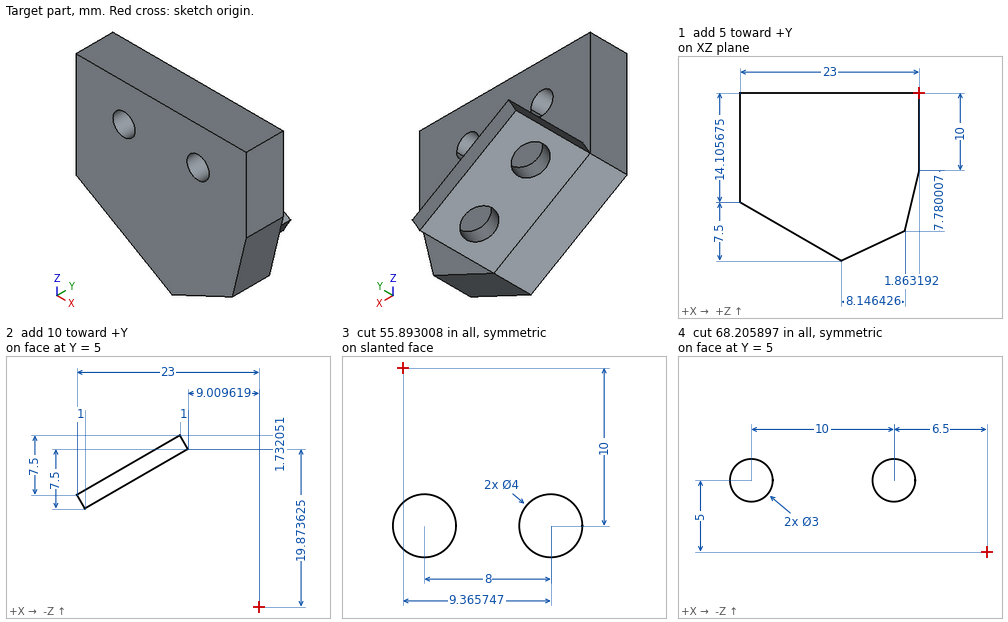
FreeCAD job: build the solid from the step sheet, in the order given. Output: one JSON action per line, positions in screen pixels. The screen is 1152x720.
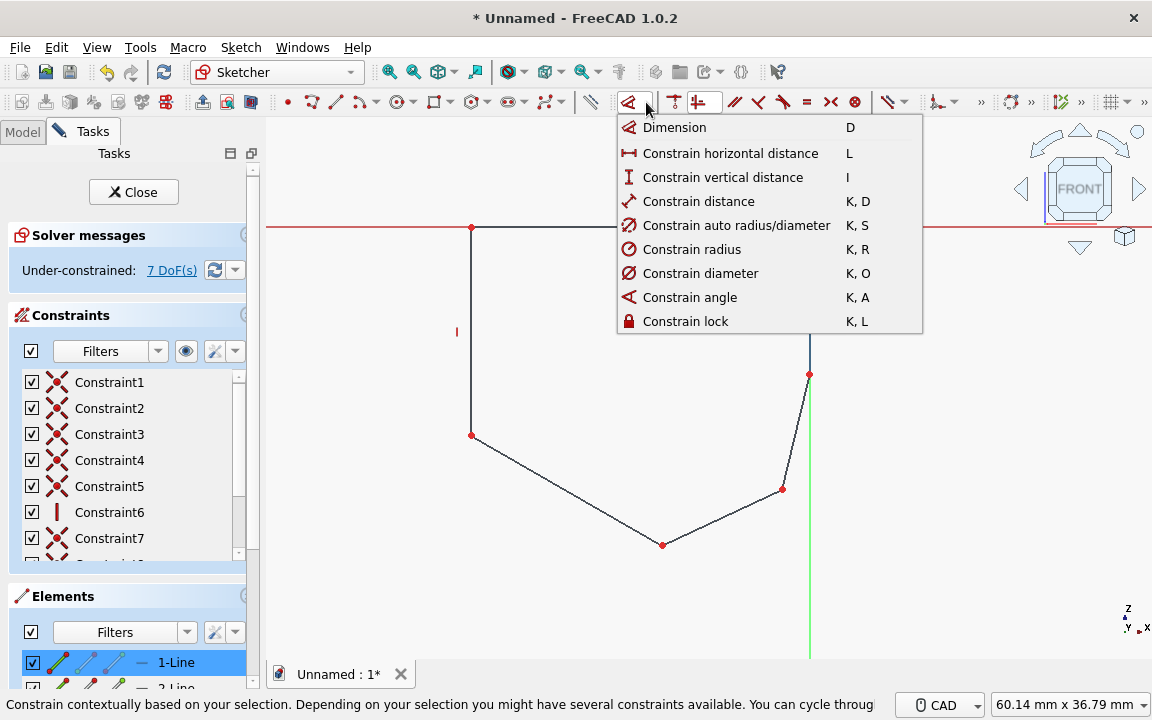
{"action": "left_click", "coordinate": [770, 177]}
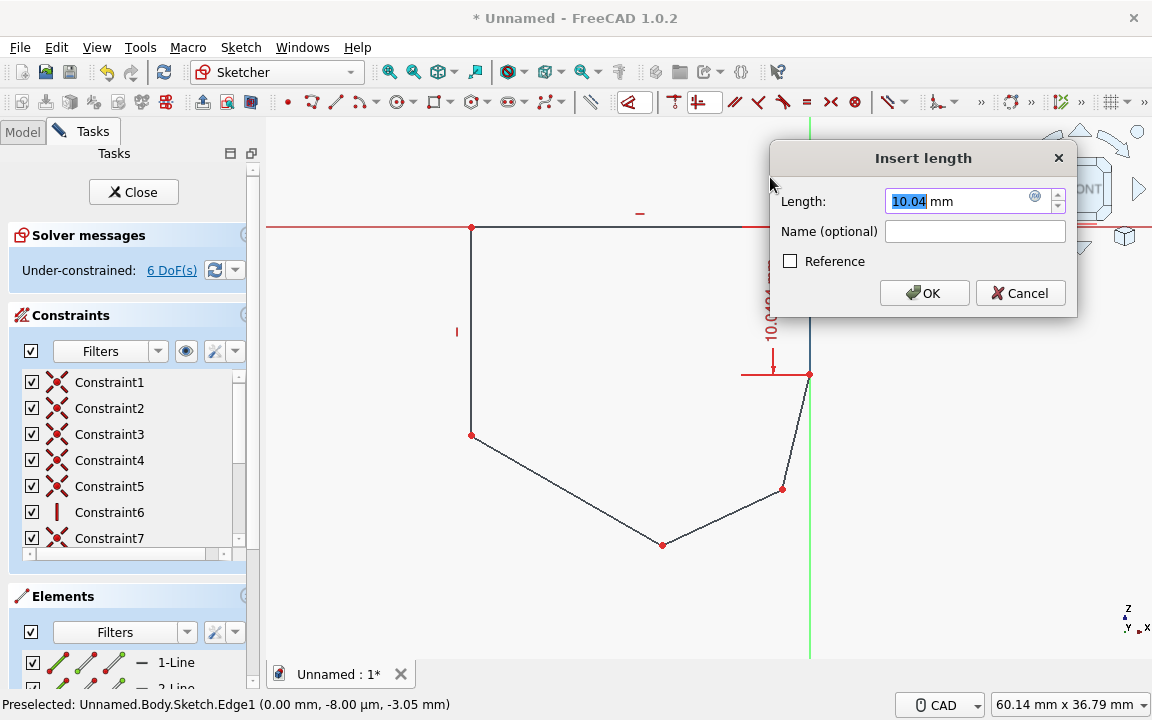
{"action": "type", "text": "10"}
{"action": "key", "text": "Return"}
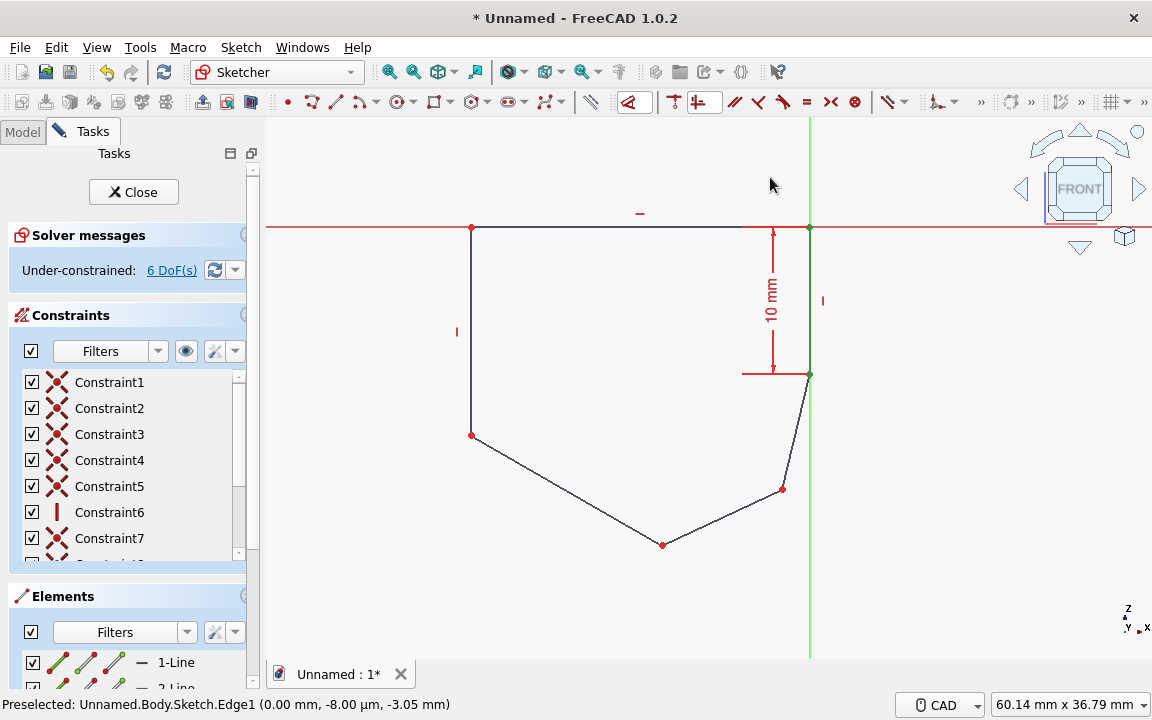
{"action": "left_click", "coordinate": [573, 227]}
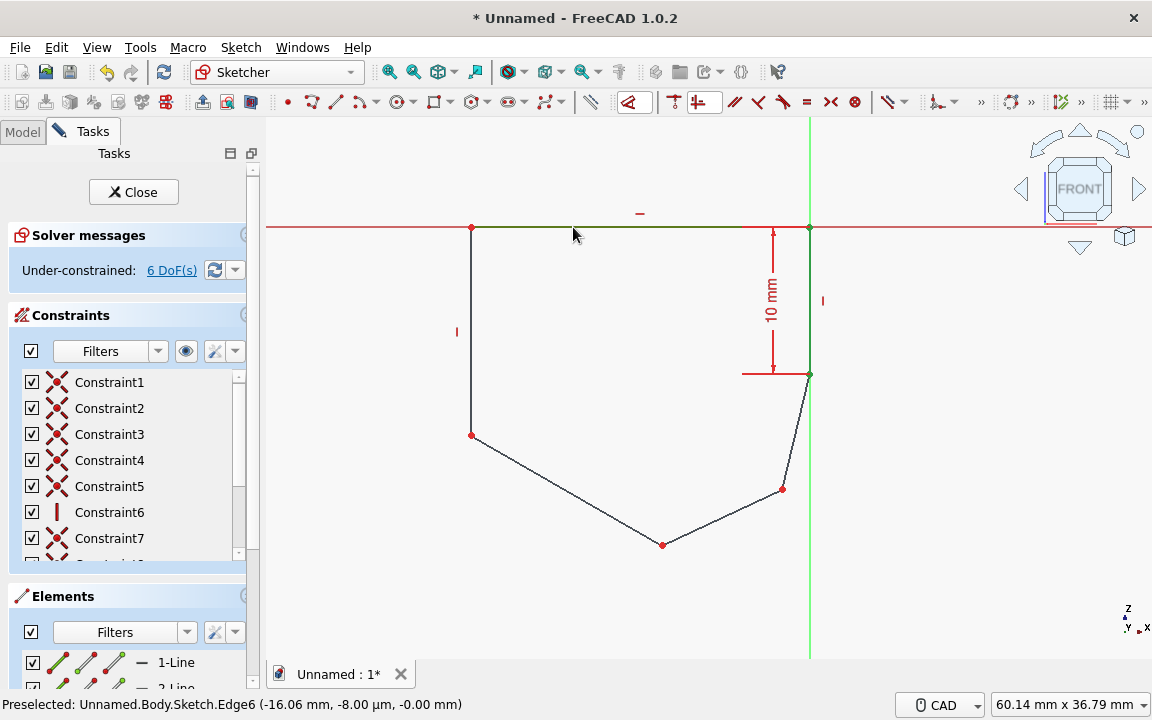
{"action": "key", "text": "l"}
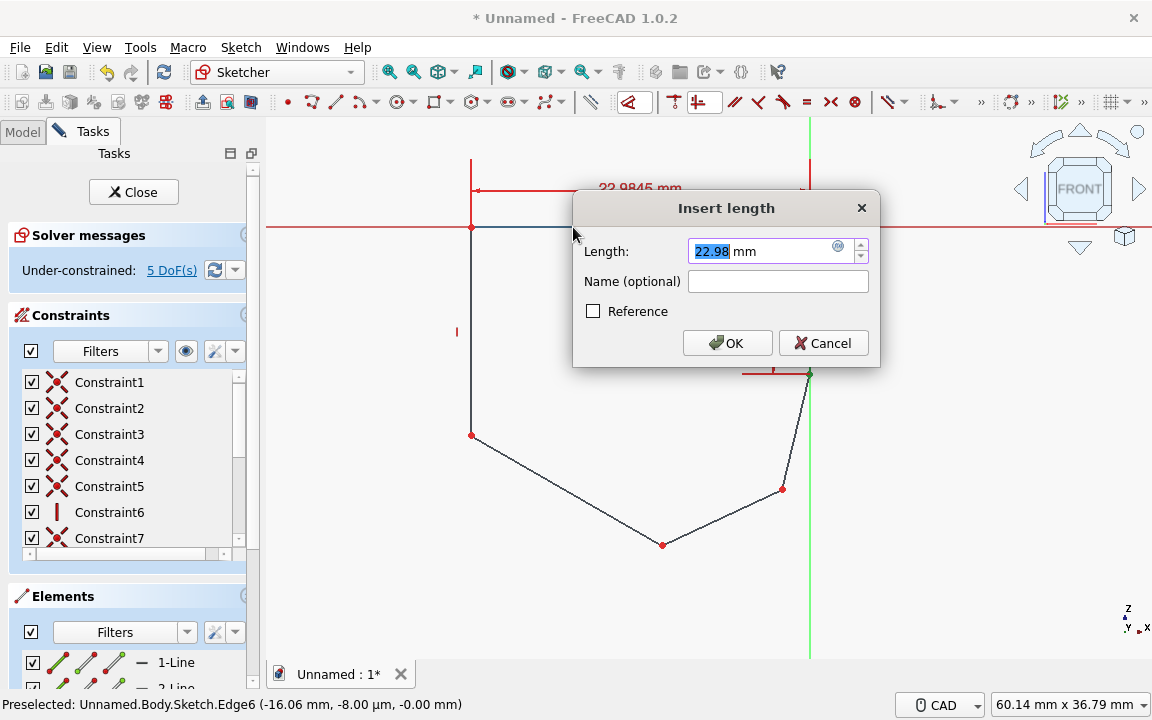
{"action": "type", "text": "23"}
{"action": "key", "text": "Return"}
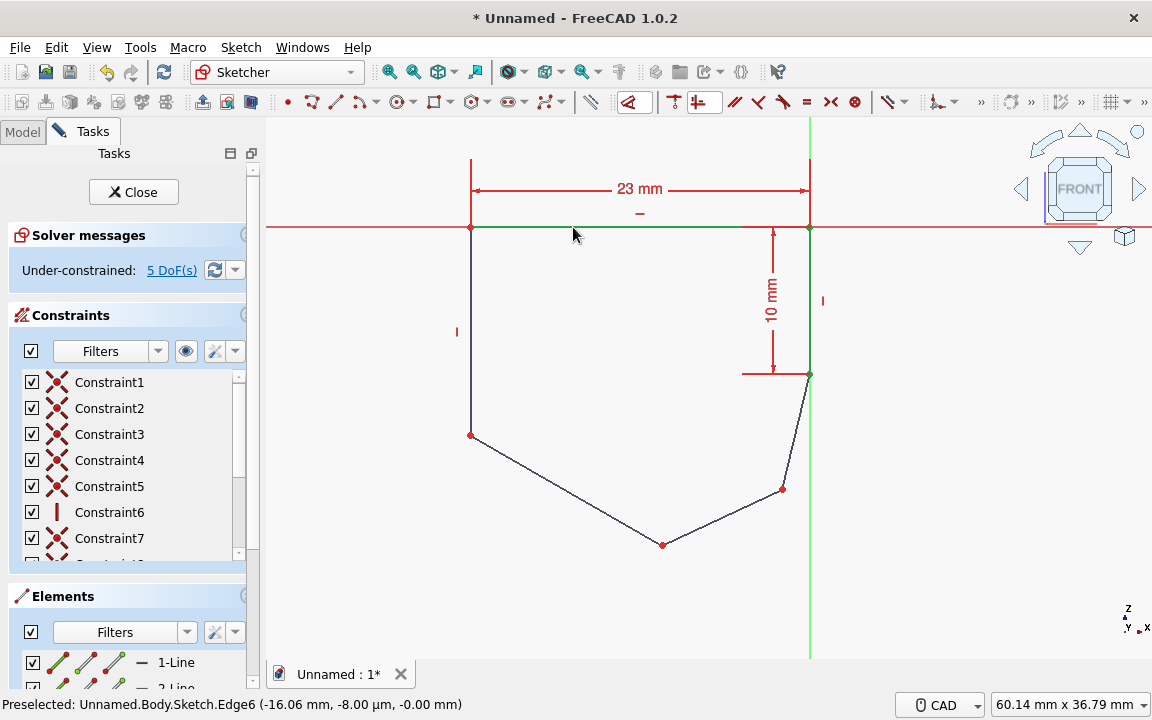
{"action": "left_click", "coordinate": [605, 513]}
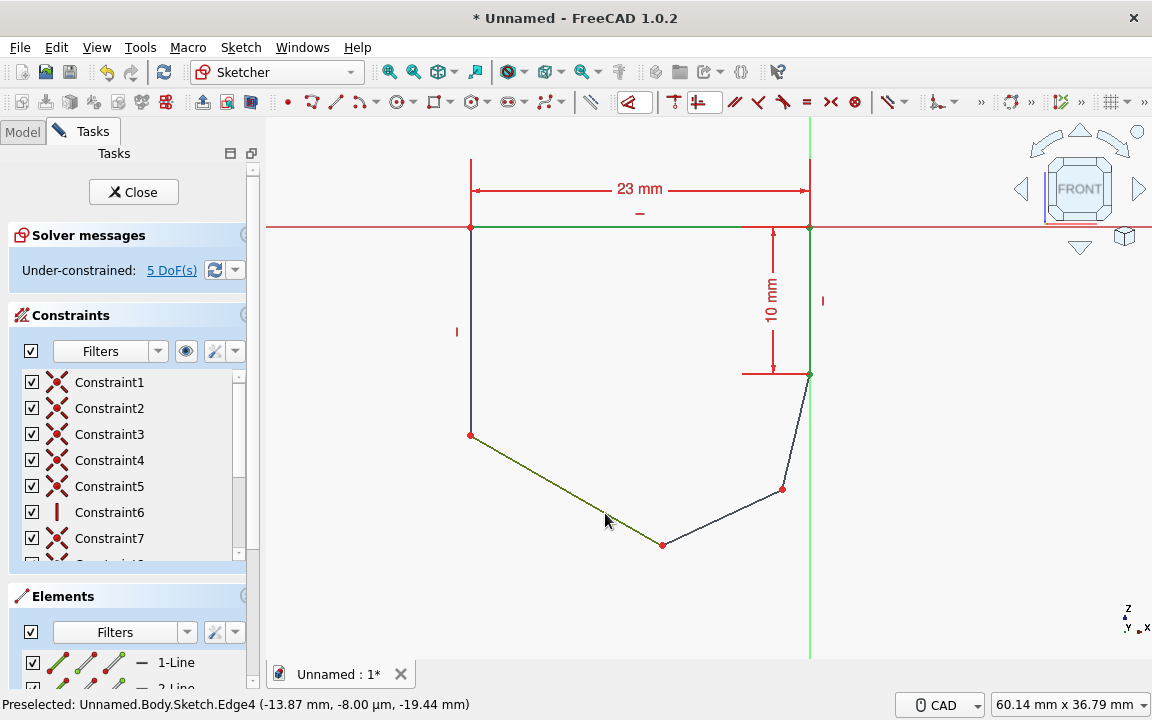
{"action": "key", "text": "i"}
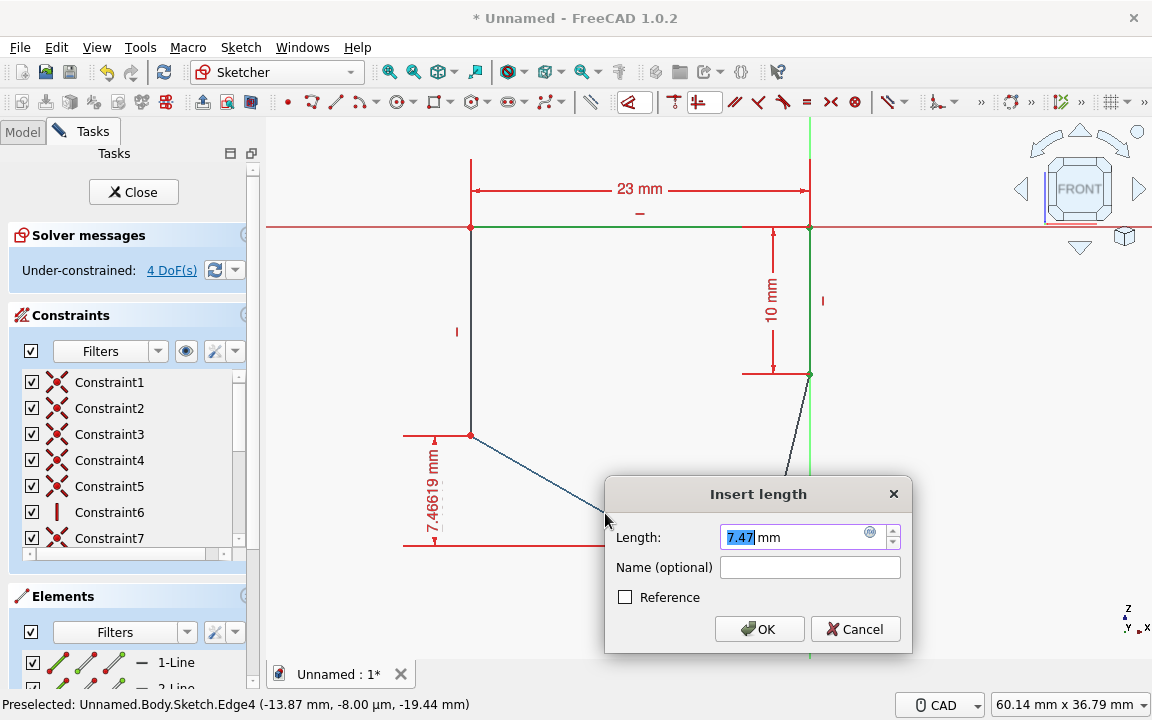
{"action": "type", "text": "7.5"}
{"action": "key", "text": "Return"}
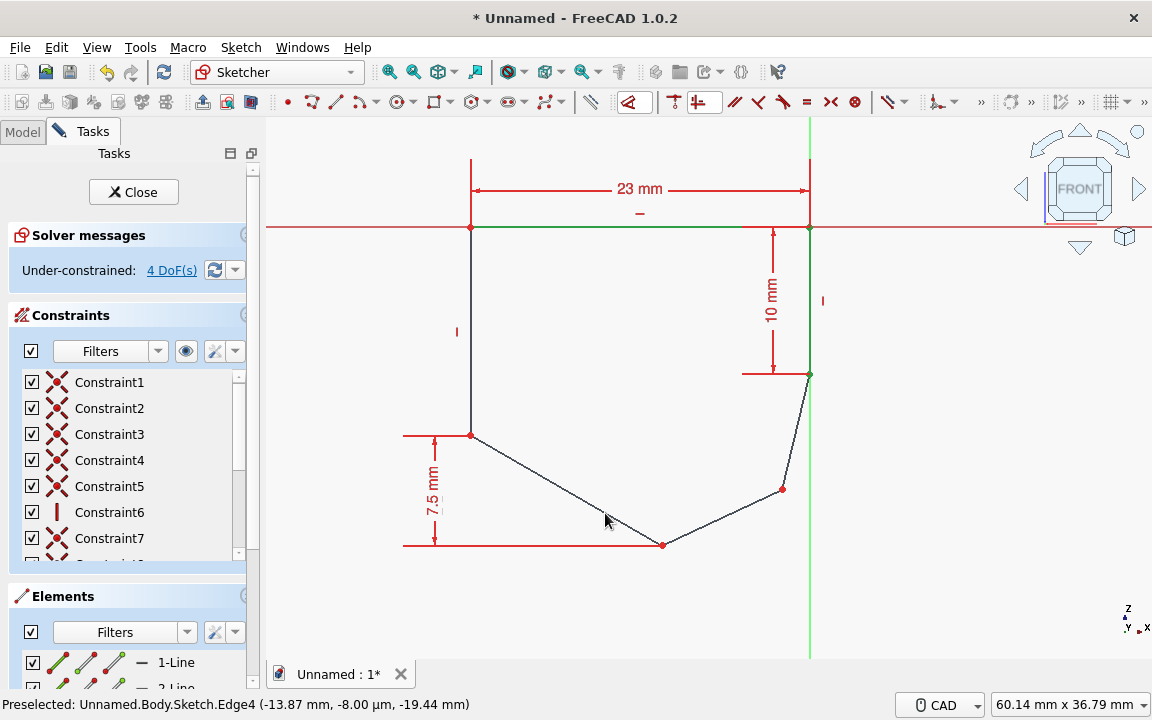
{"action": "left_click", "coordinate": [471, 373]}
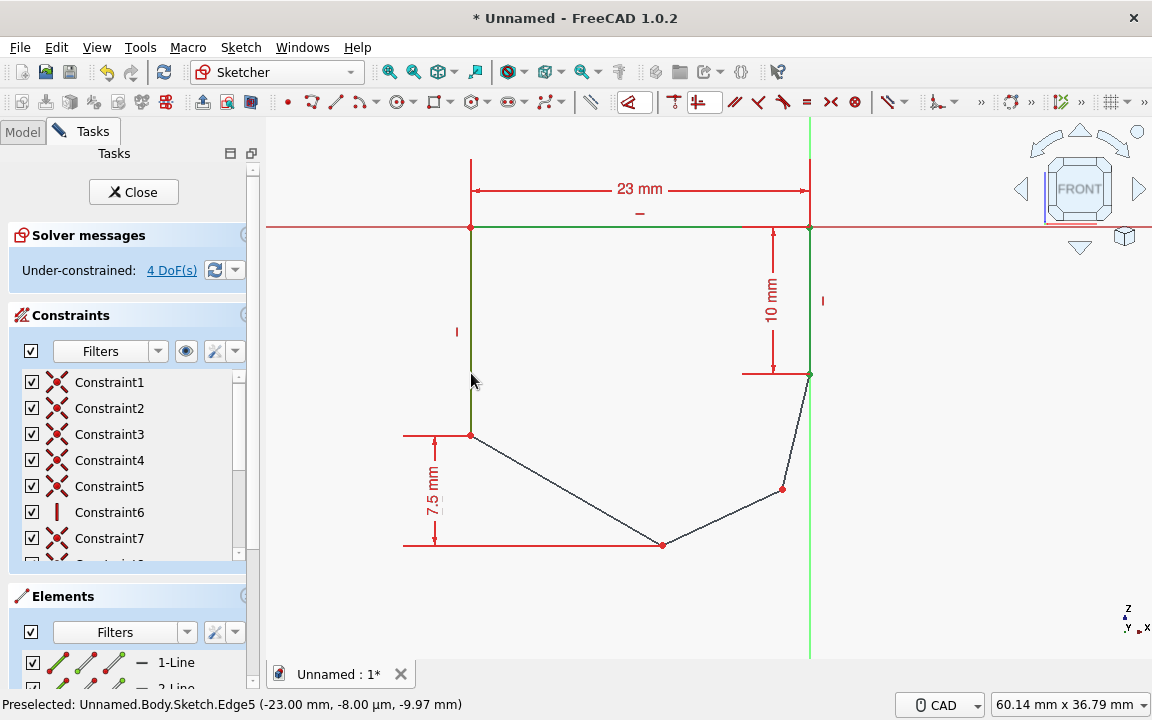
{"action": "left_click", "coordinate": [646, 102]}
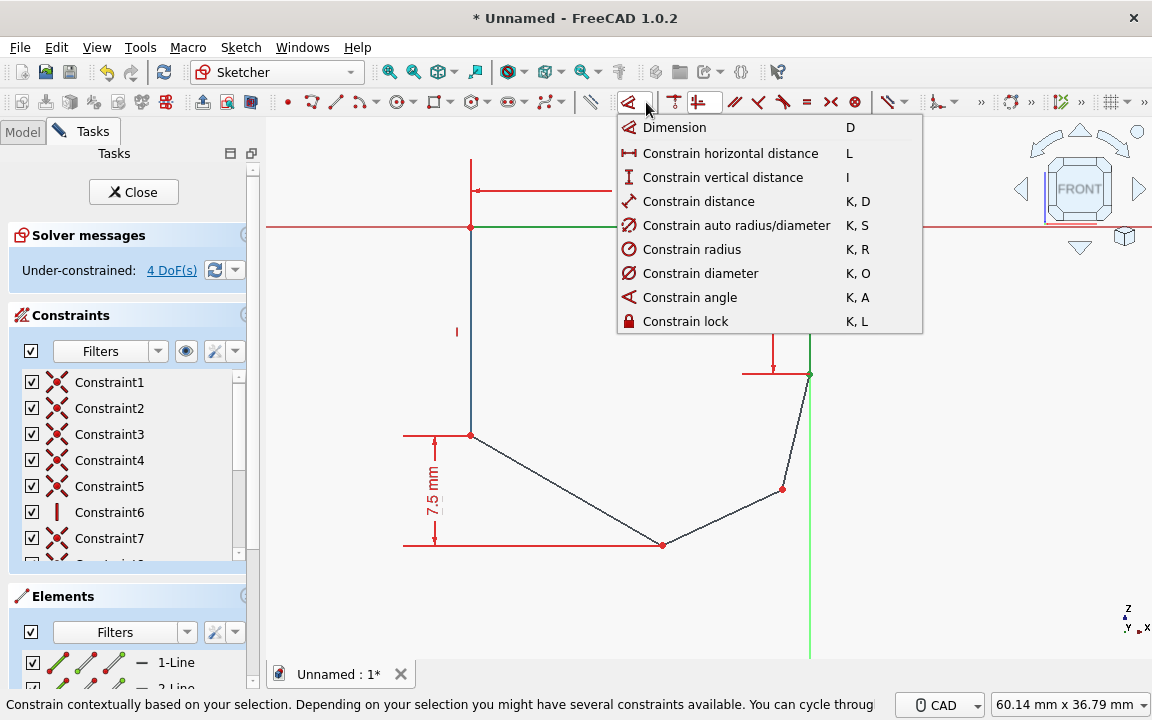
{"action": "left_click", "coordinate": [770, 177]}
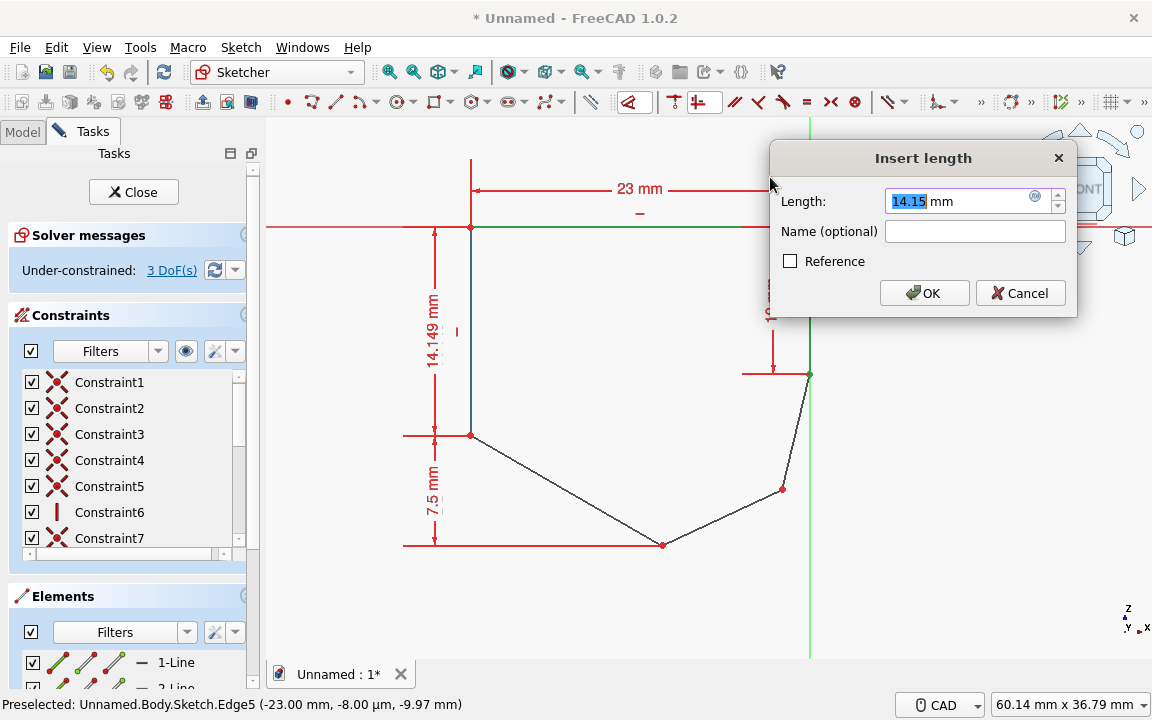
{"action": "type", "text": "14.105675"}
{"action": "key", "text": "Return"}